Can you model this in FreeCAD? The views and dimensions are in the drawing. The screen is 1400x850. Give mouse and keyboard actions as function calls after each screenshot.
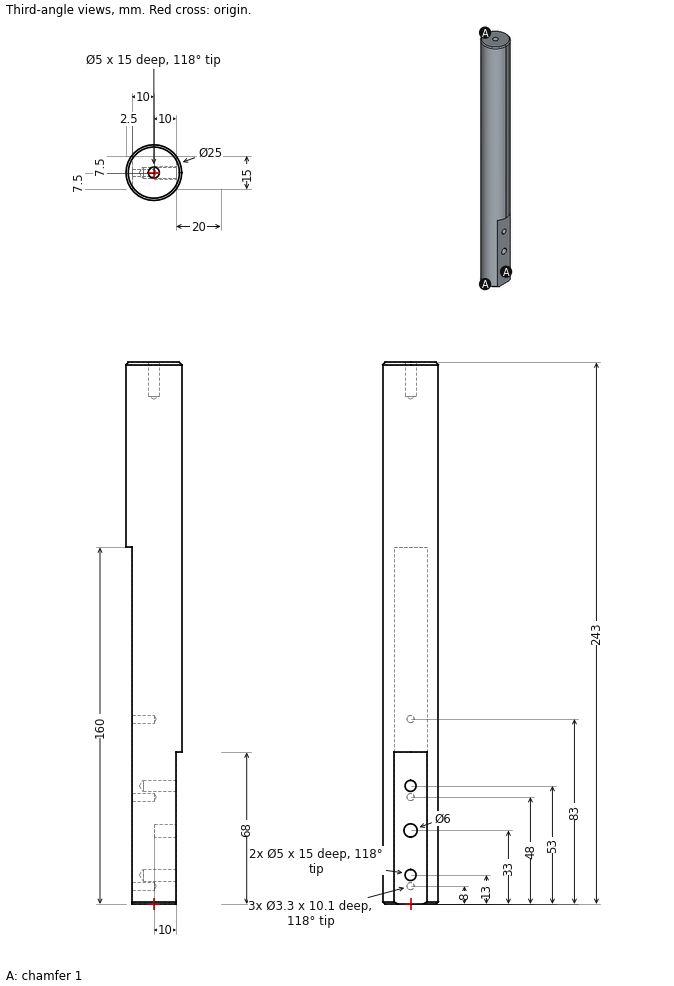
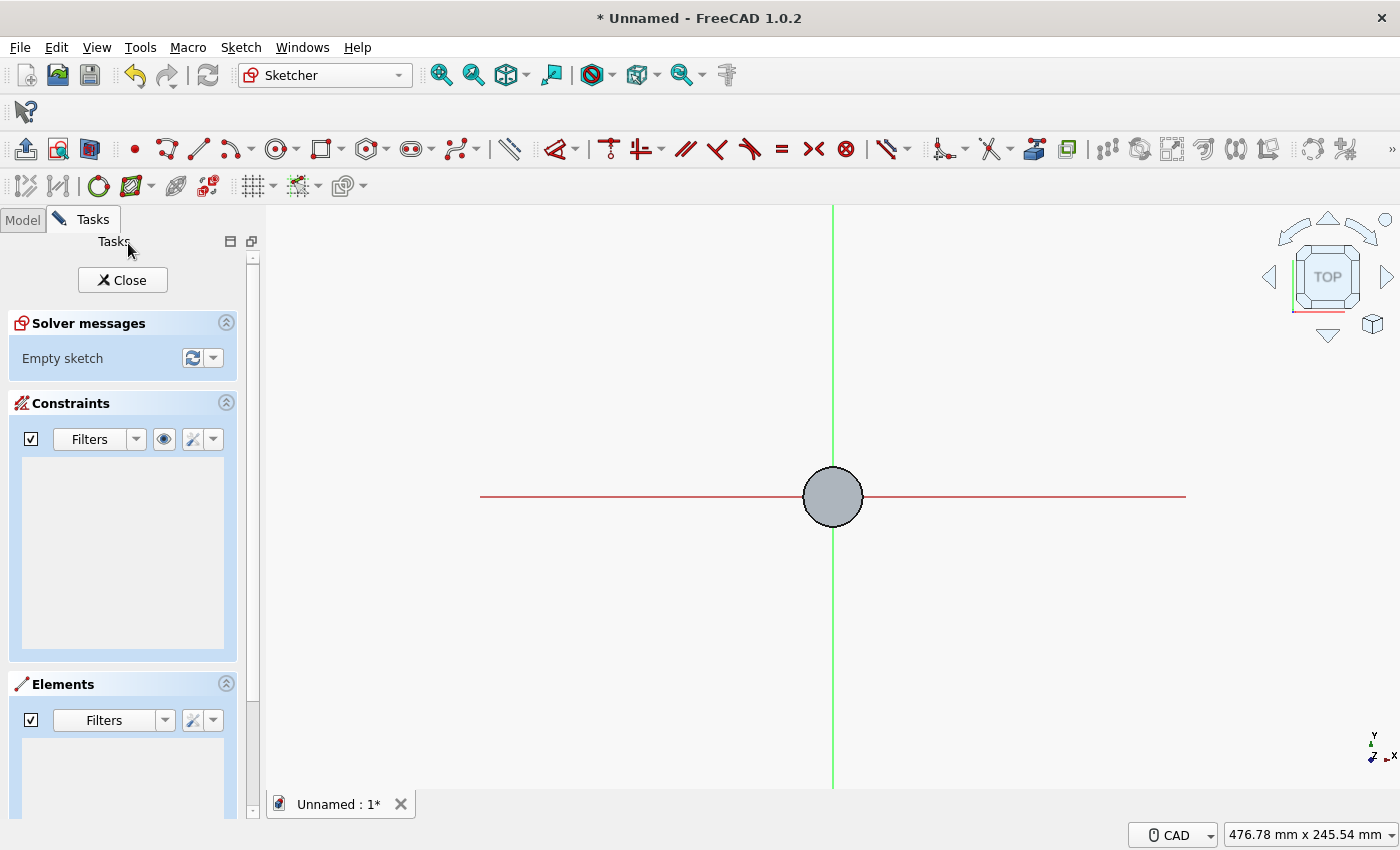
key(q)
key(s)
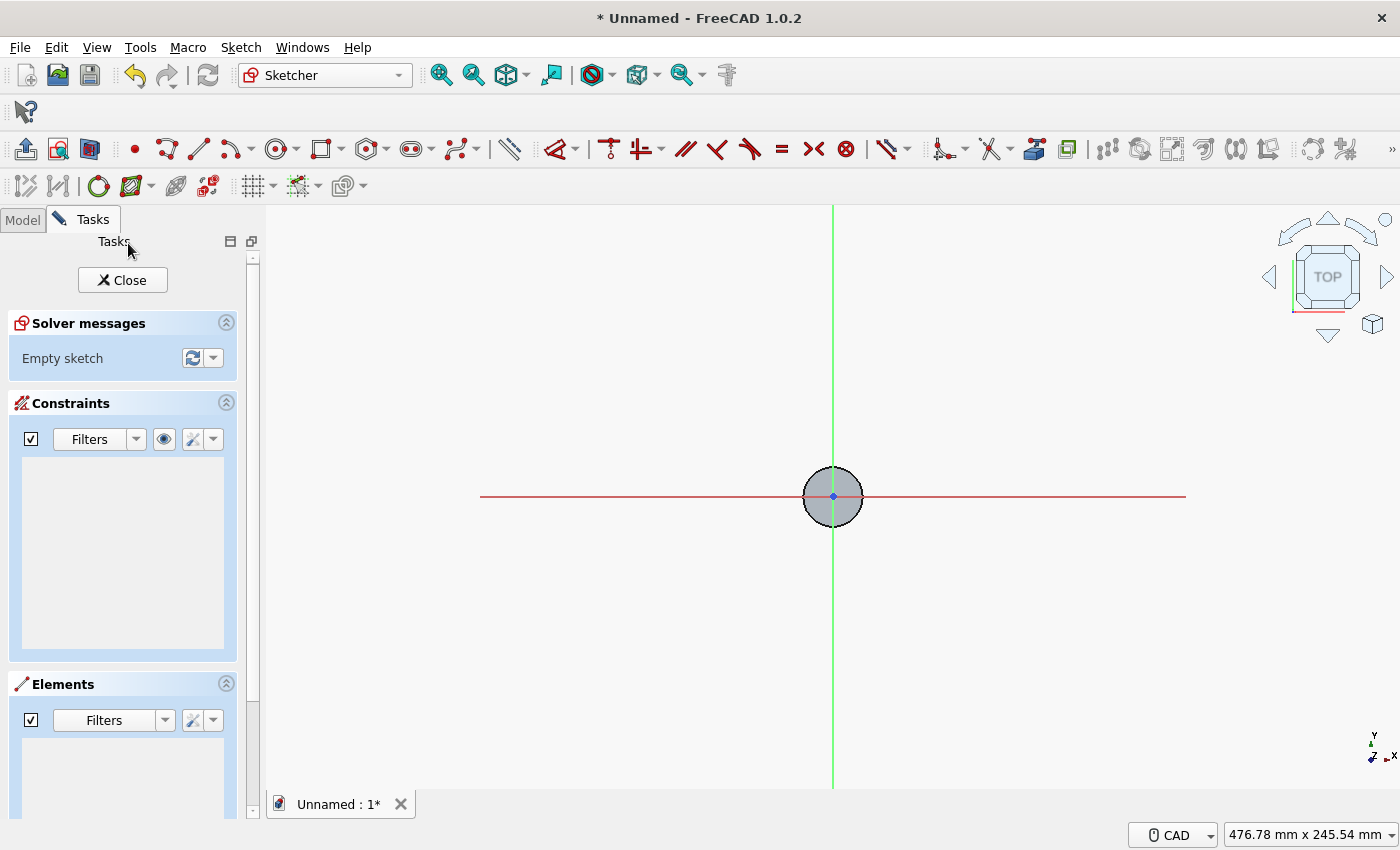
scroll(882, 497, up, 11)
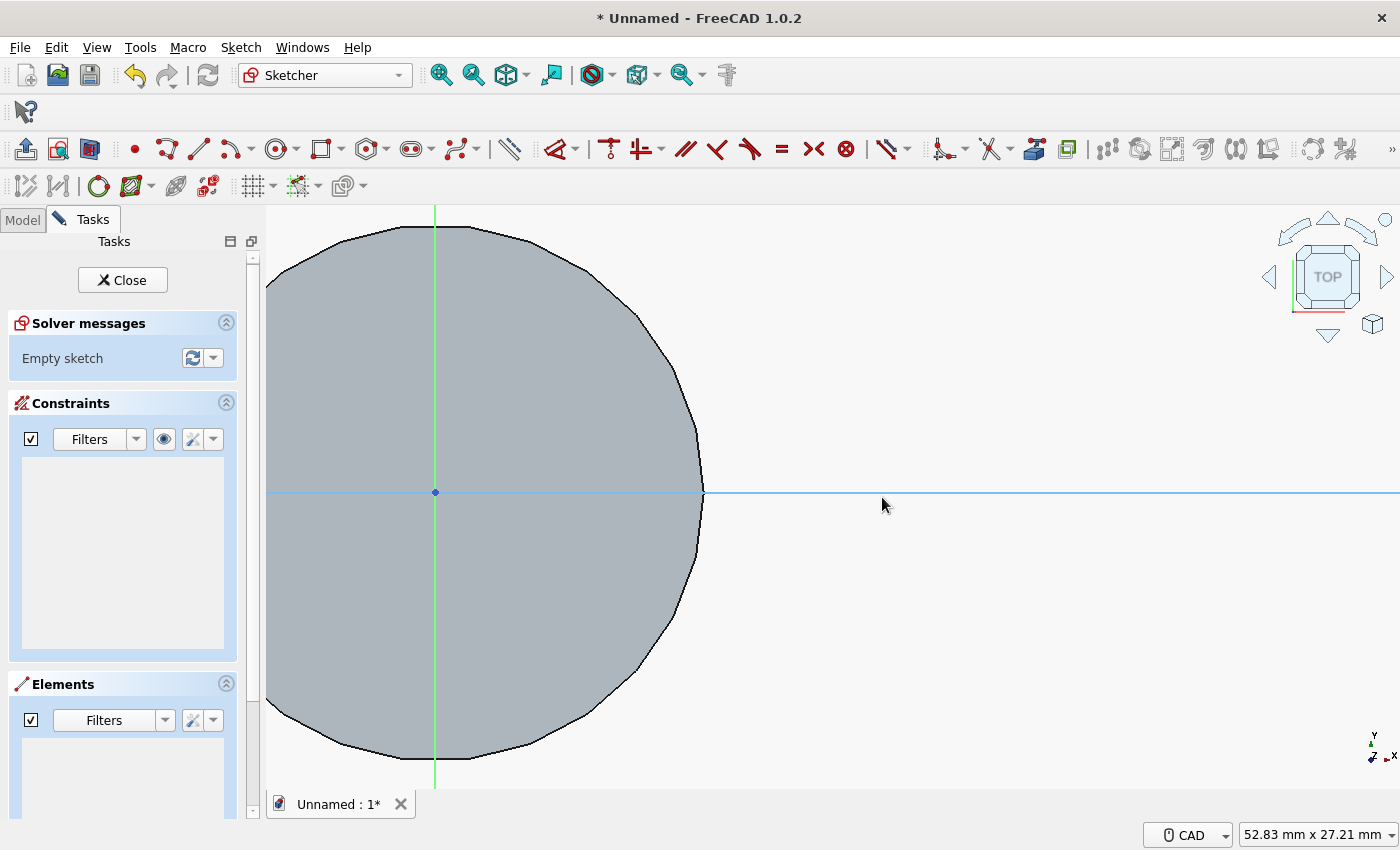
key(g)
key(r)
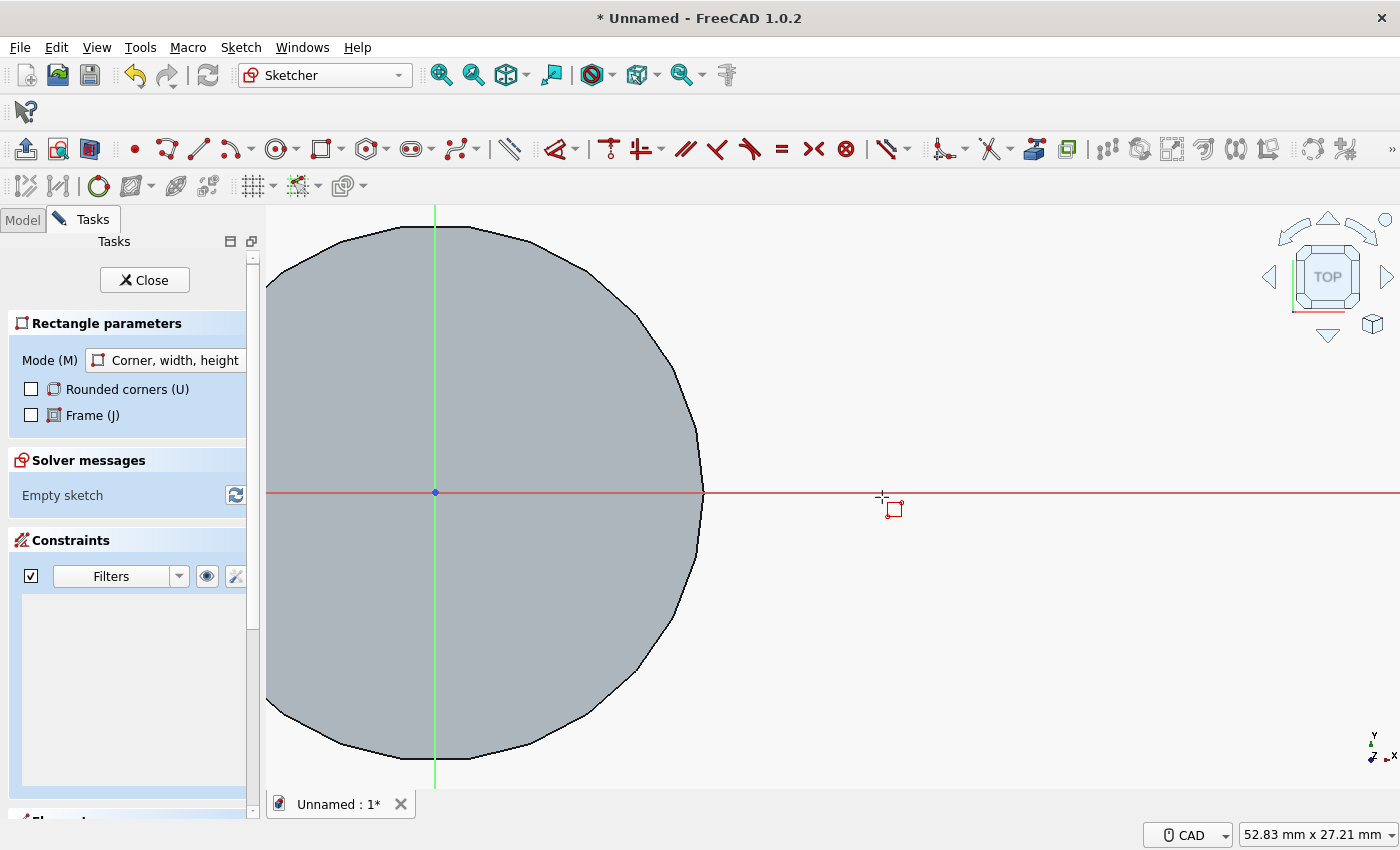
click(650, 332)
click(1079, 654)
key(Escape)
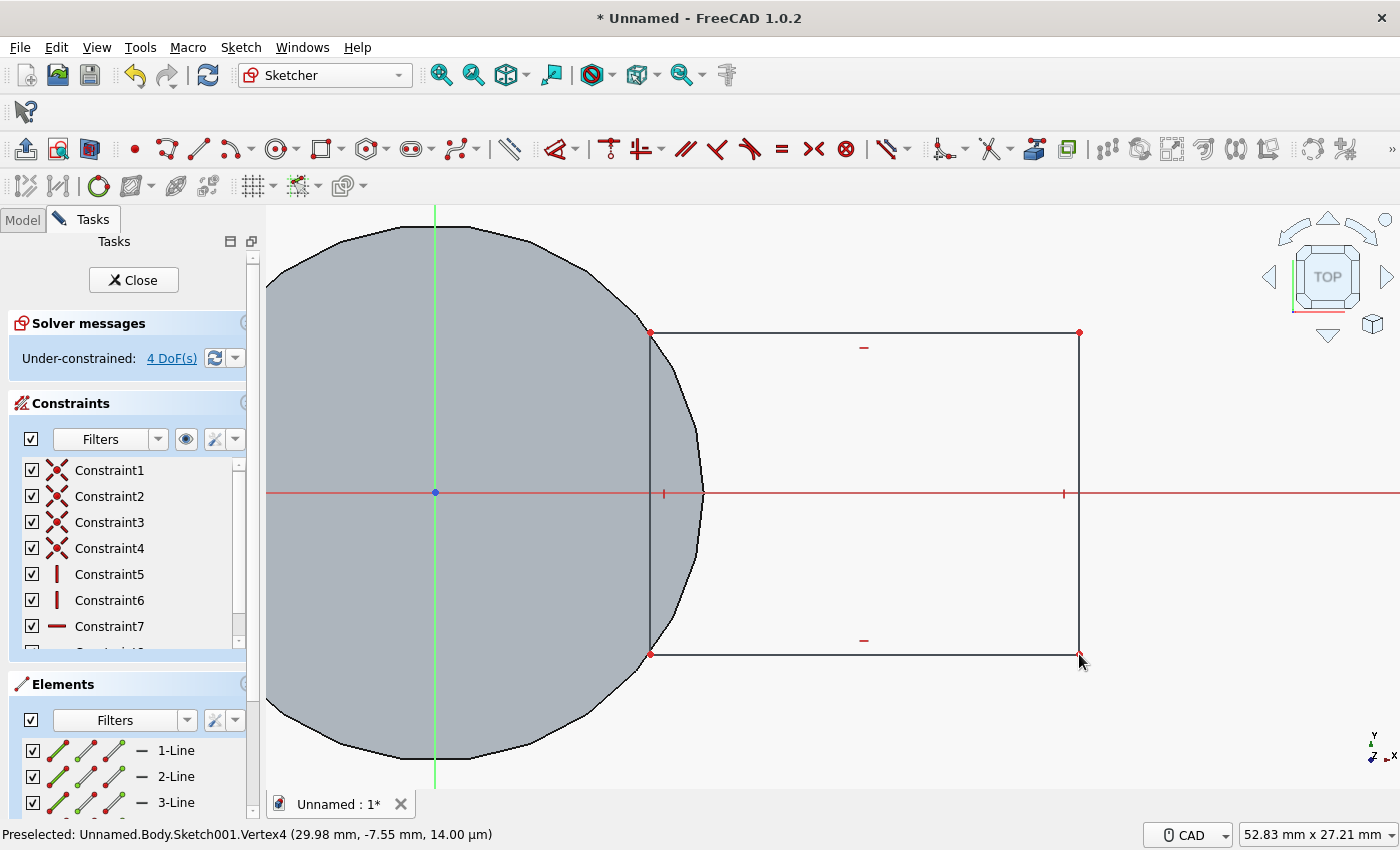
key(d)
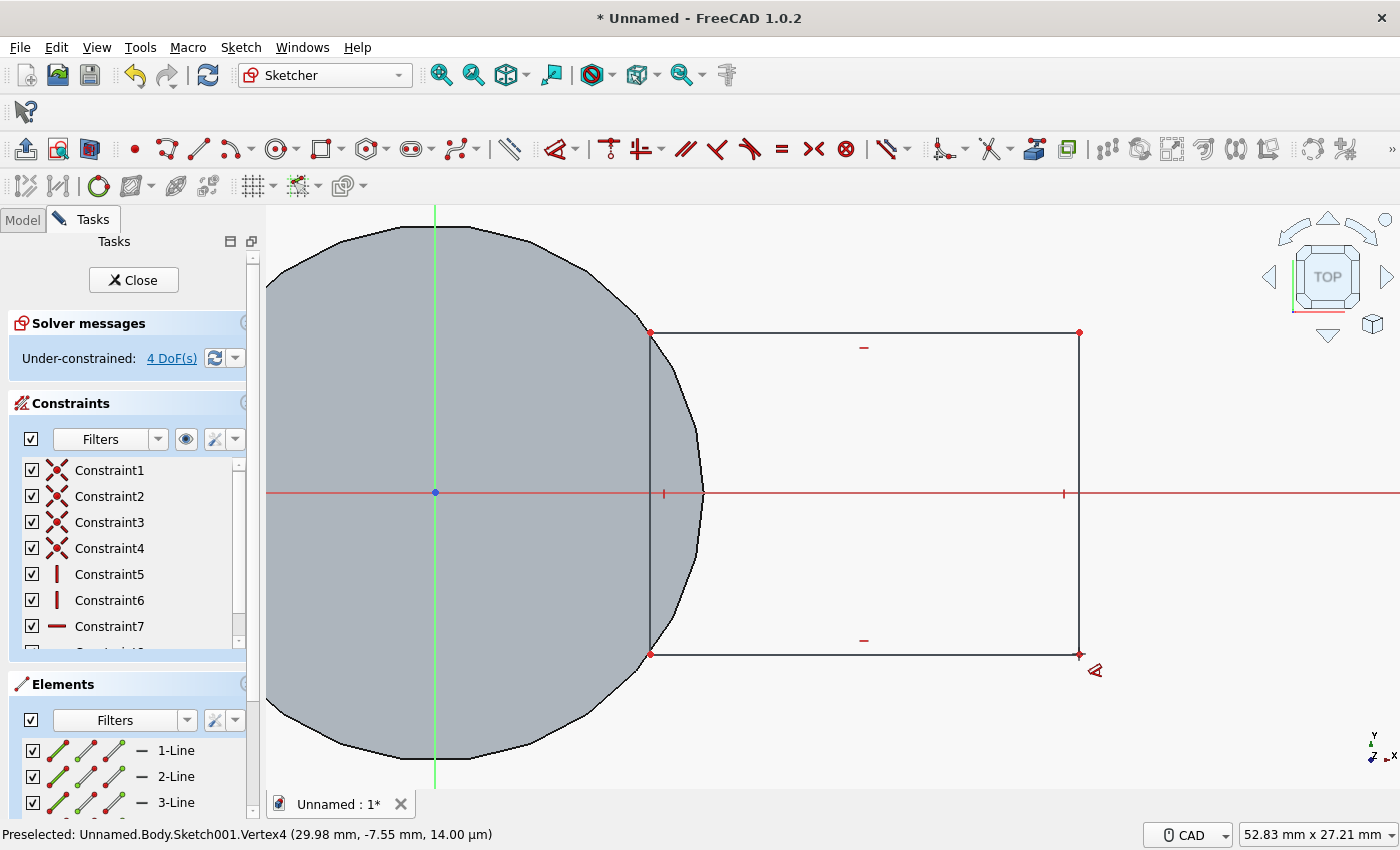
click(650, 430)
click(616, 420)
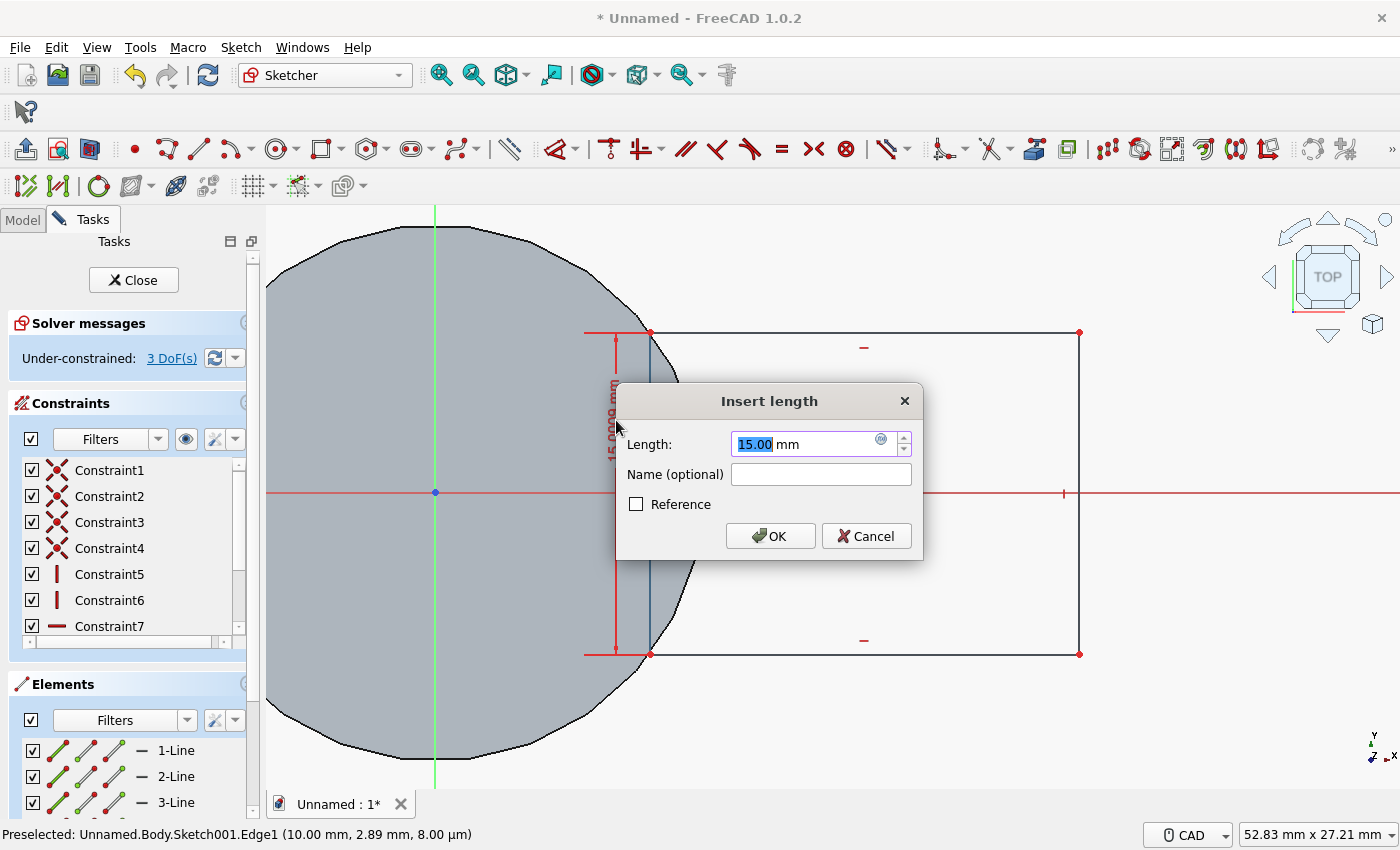
text(15)
key(Return)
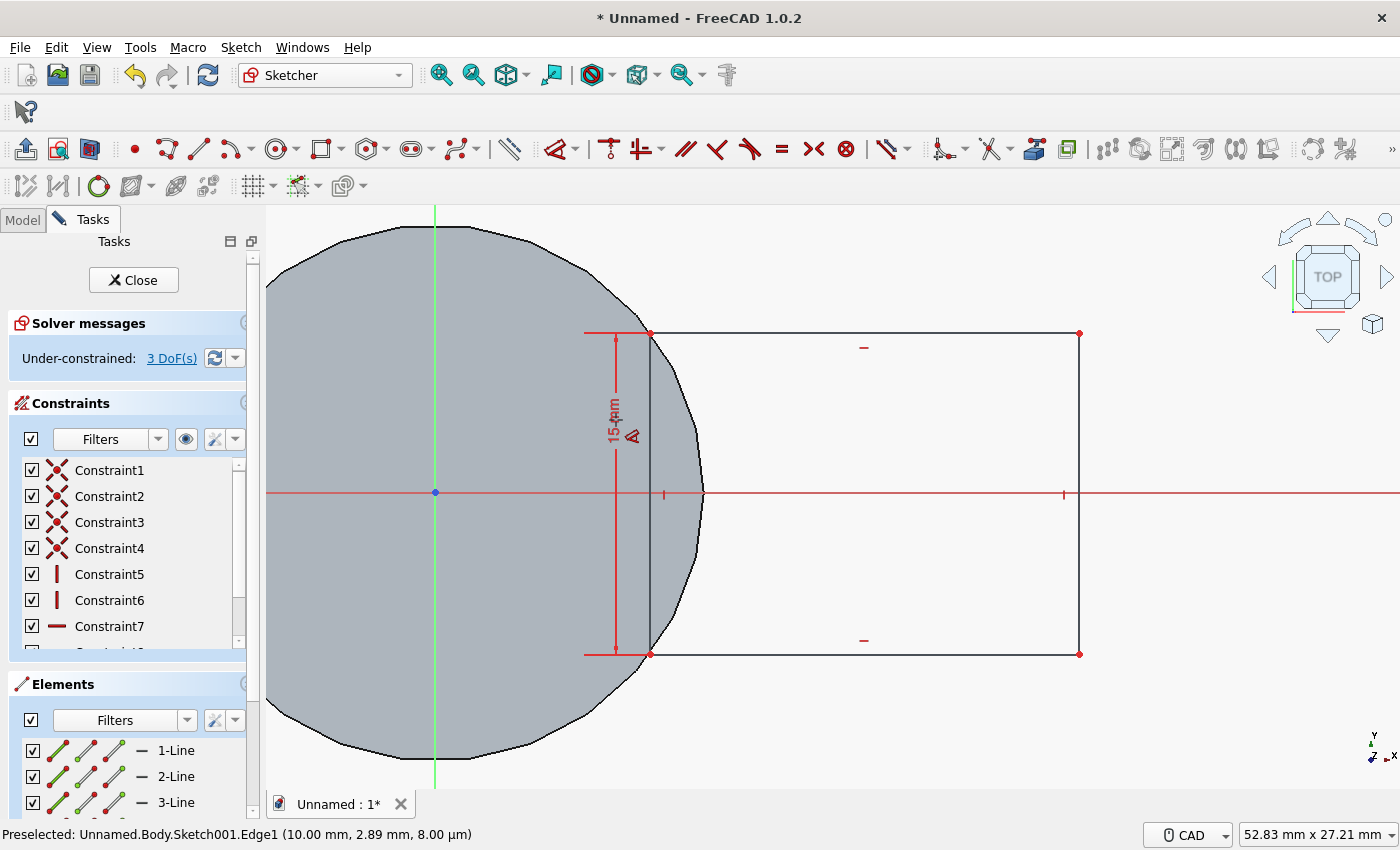
click(779, 655)
click(864, 689)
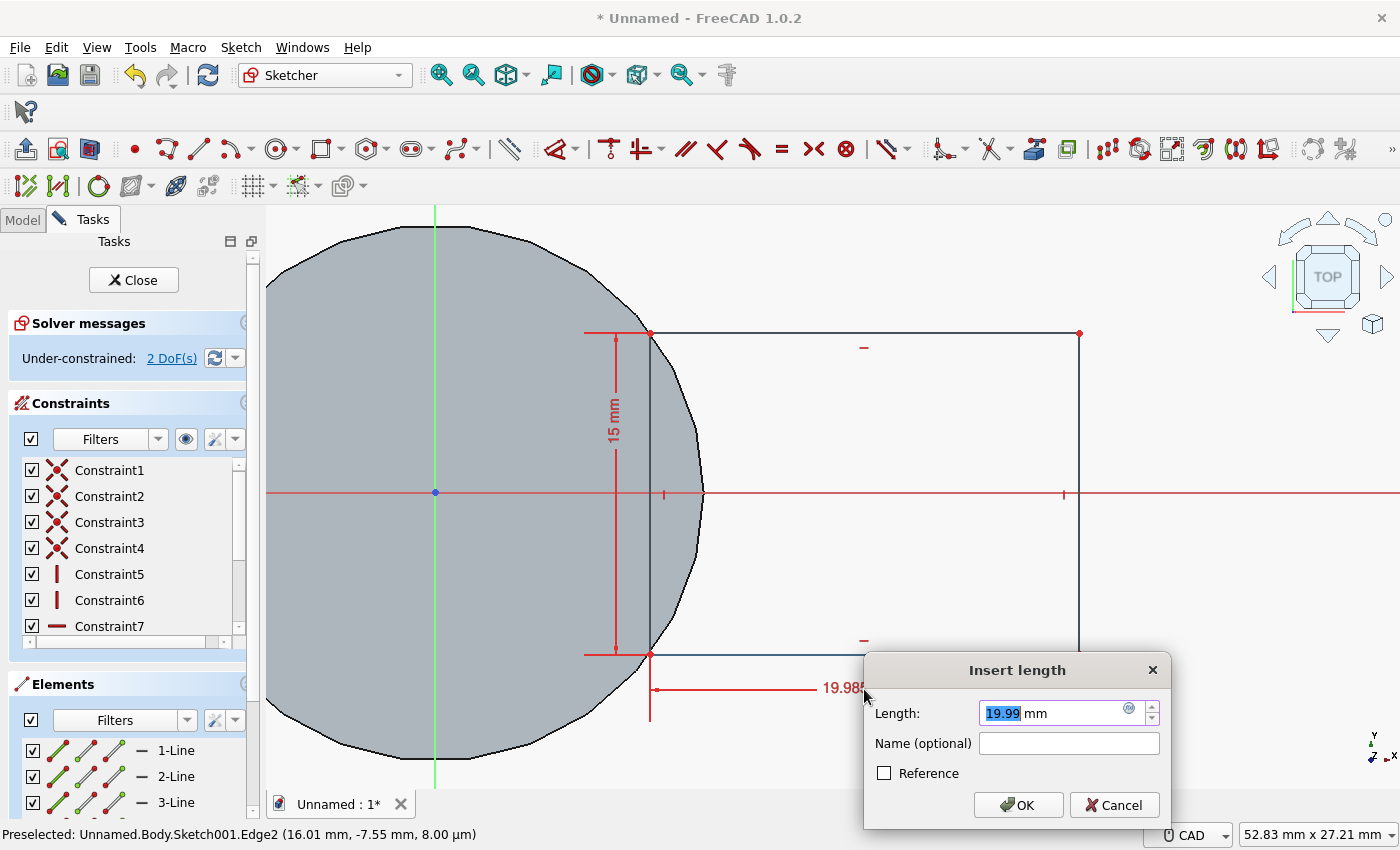
text(20)
key(Return)